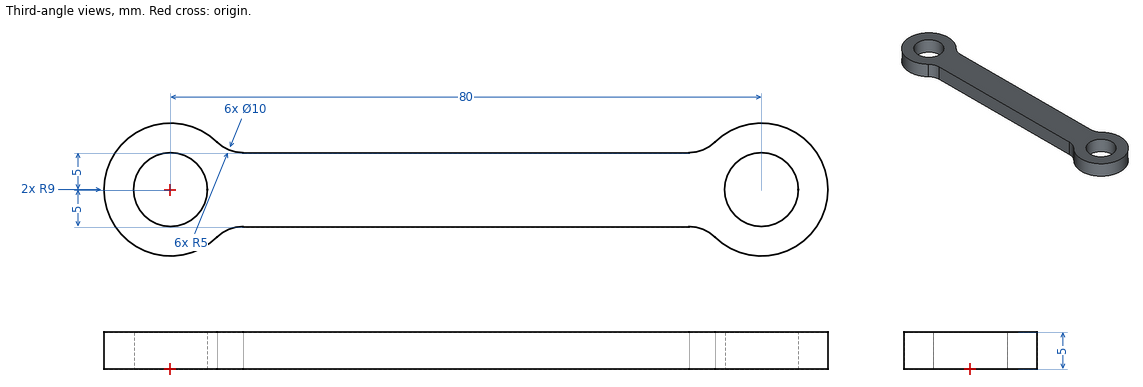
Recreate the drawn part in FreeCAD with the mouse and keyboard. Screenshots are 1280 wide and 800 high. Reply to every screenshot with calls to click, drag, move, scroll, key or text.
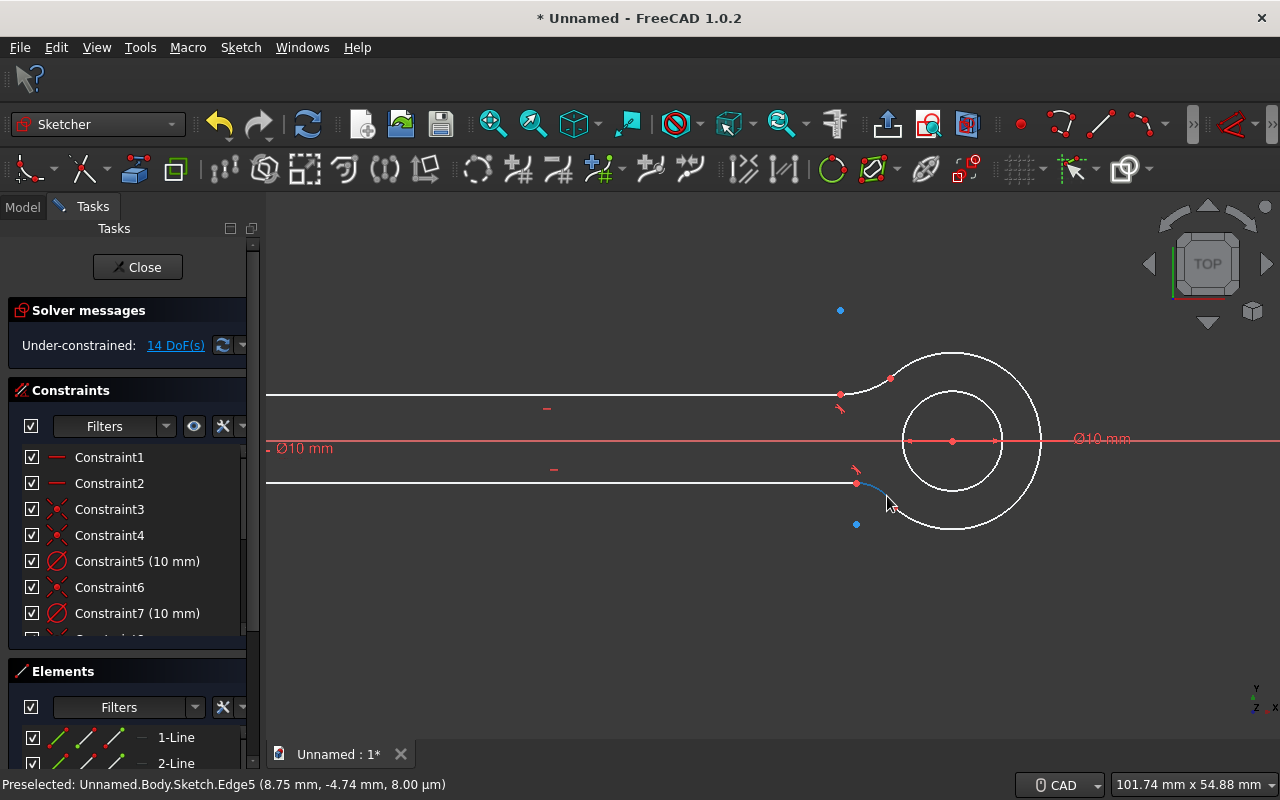
click(887, 496)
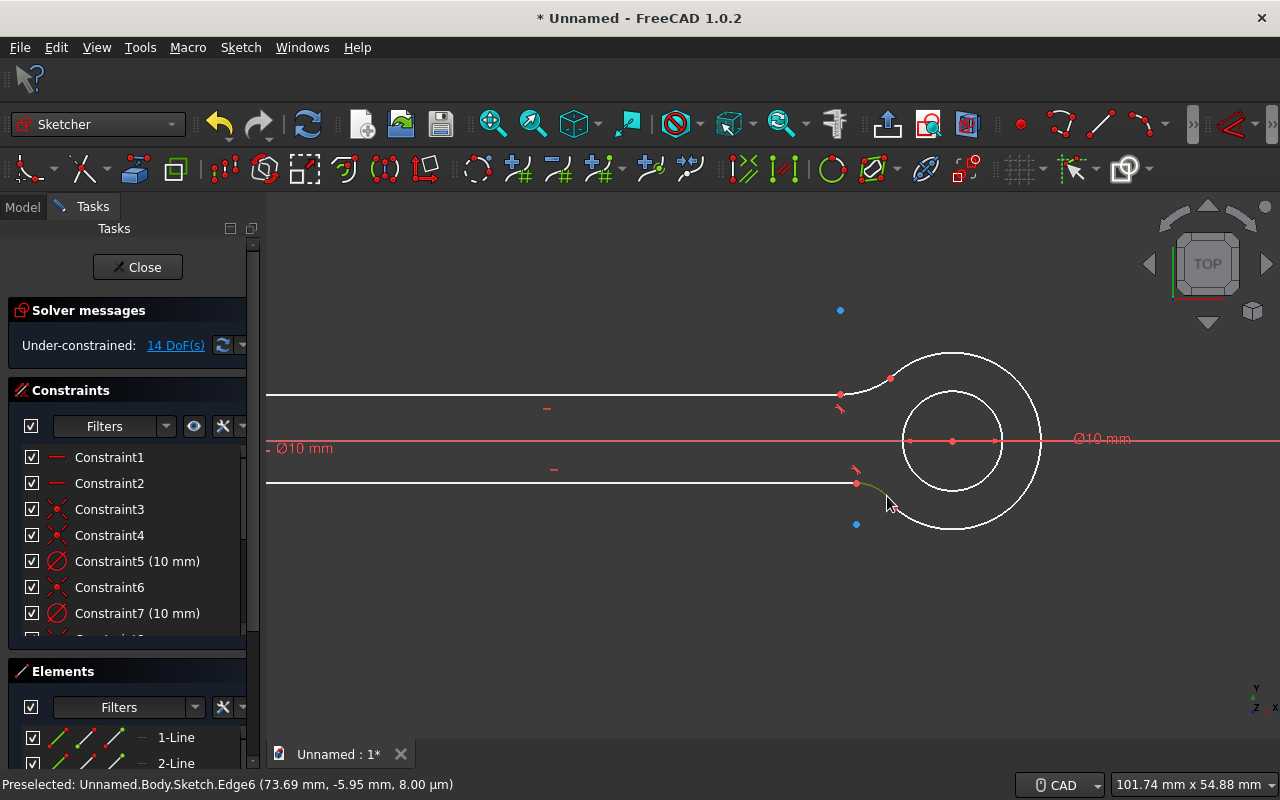
click(1008, 510)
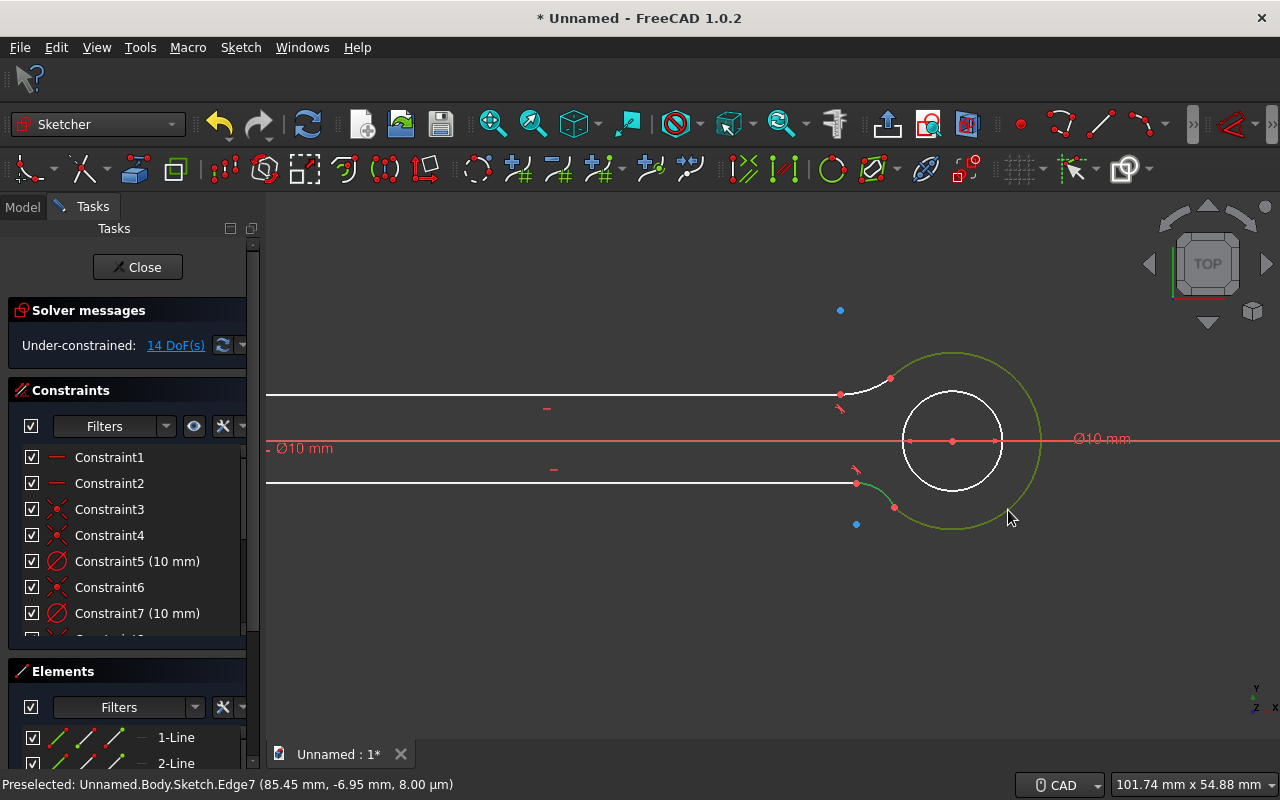
key(t)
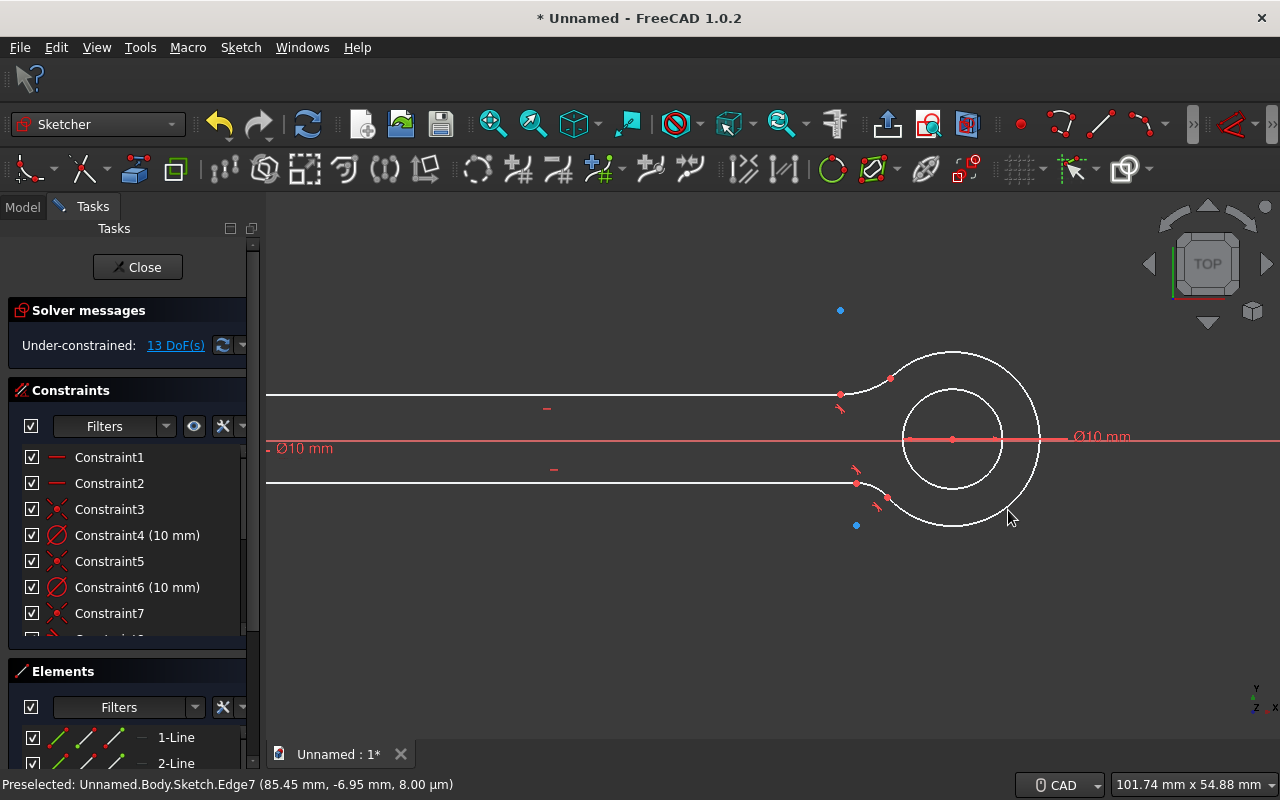
click(1001, 511)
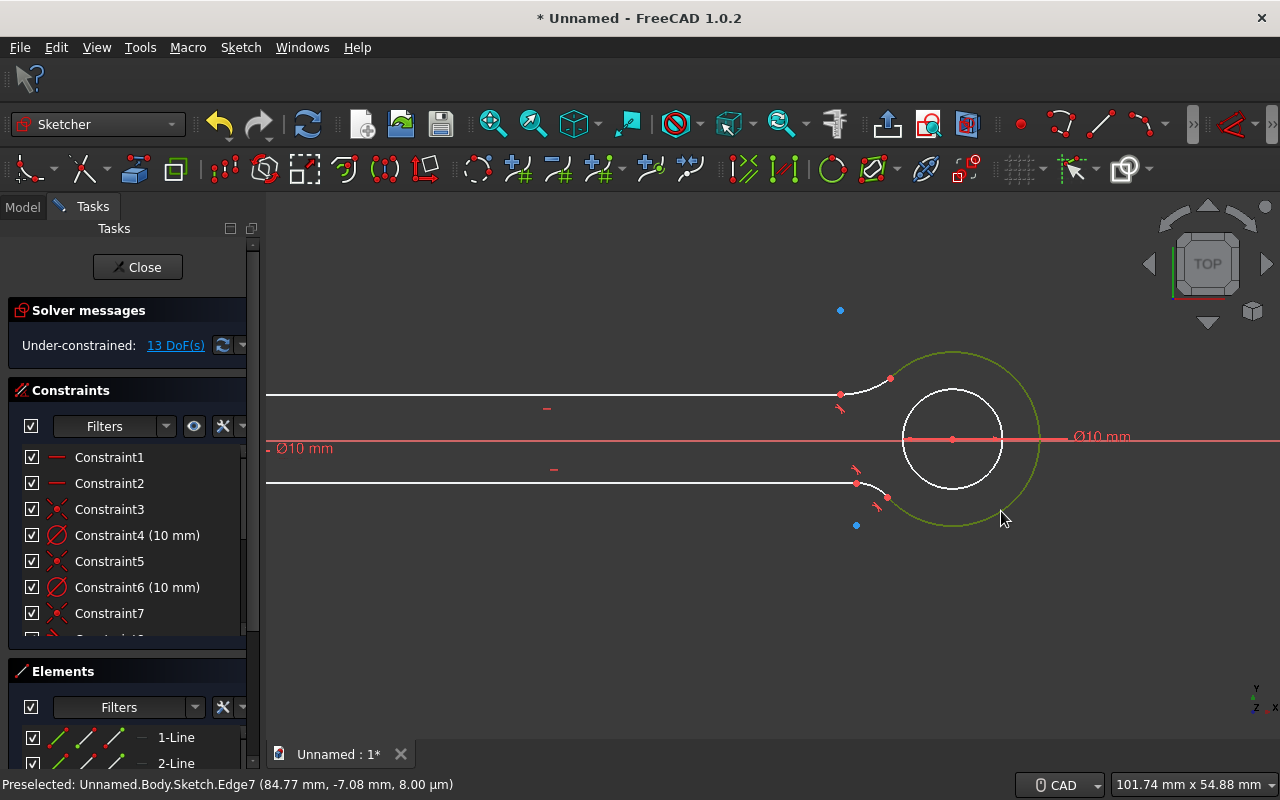
click(857, 393)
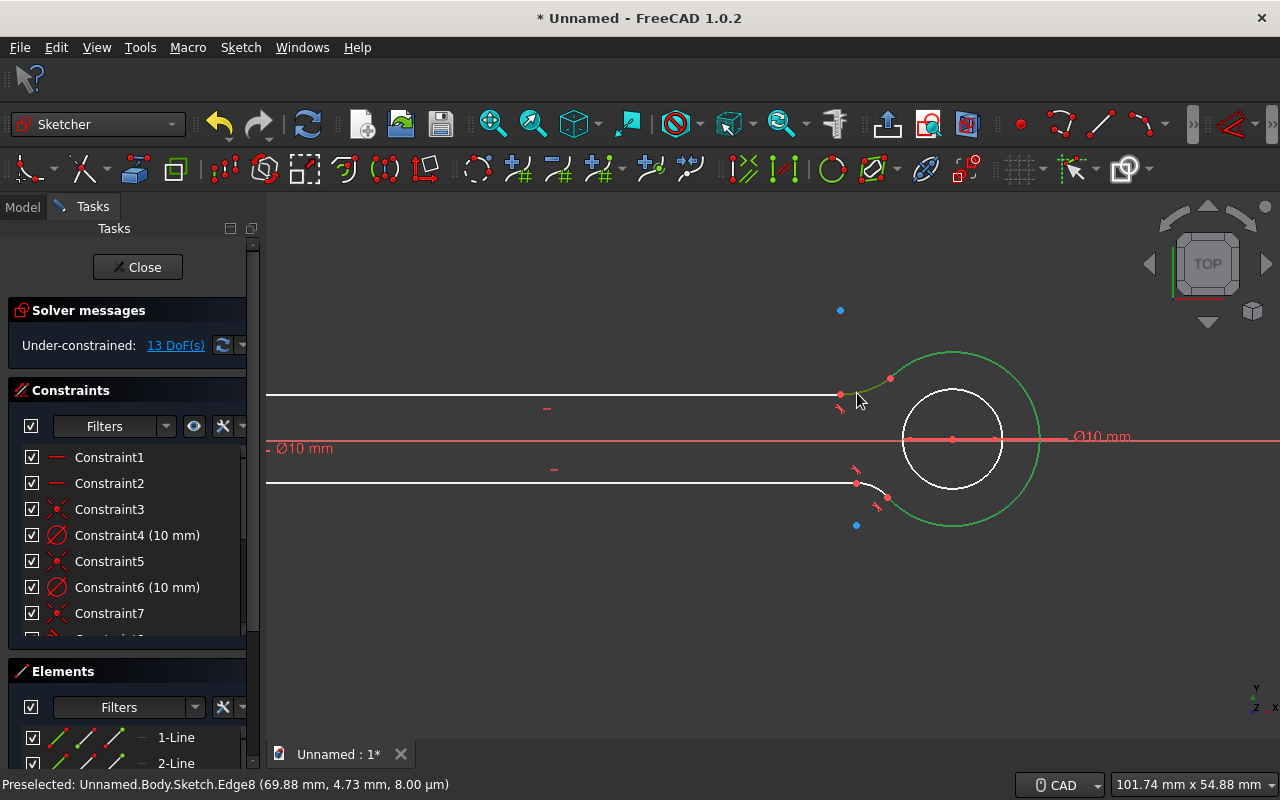
key(t)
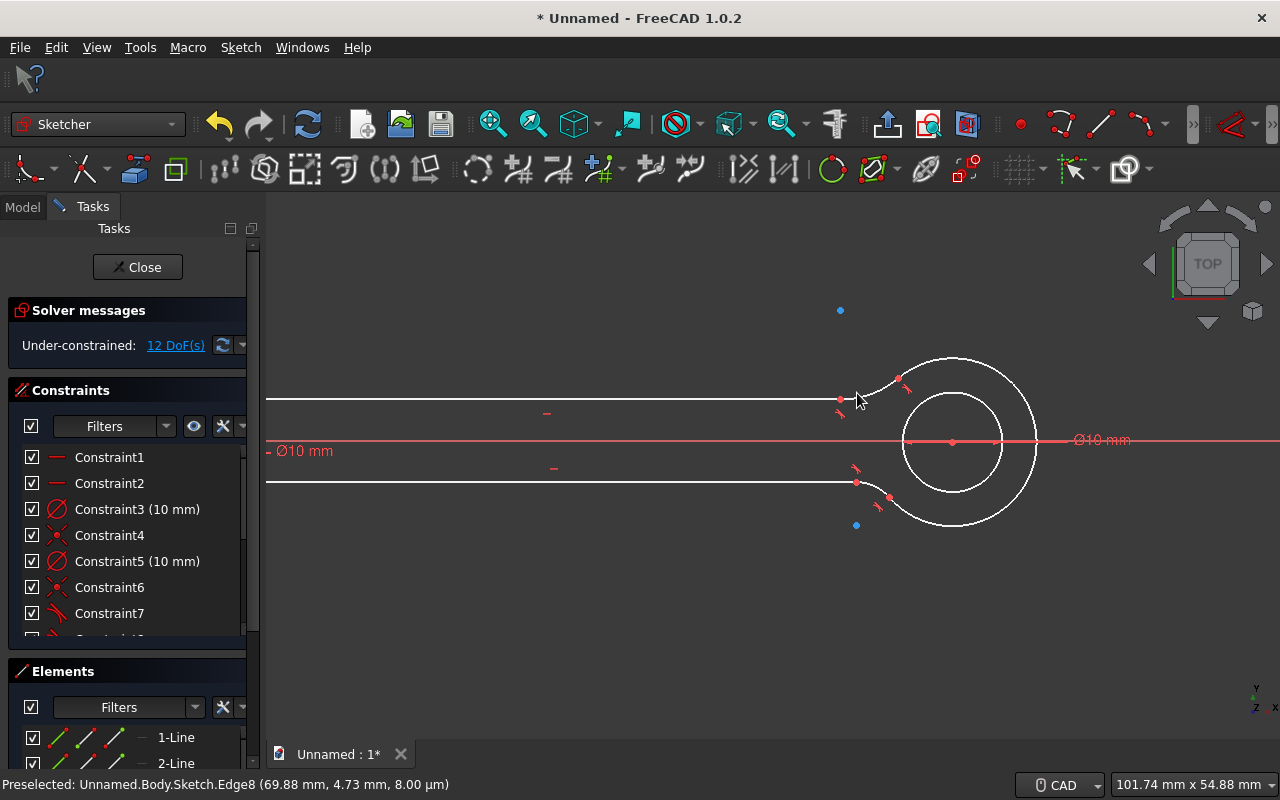
scroll(887, 495, down, 3)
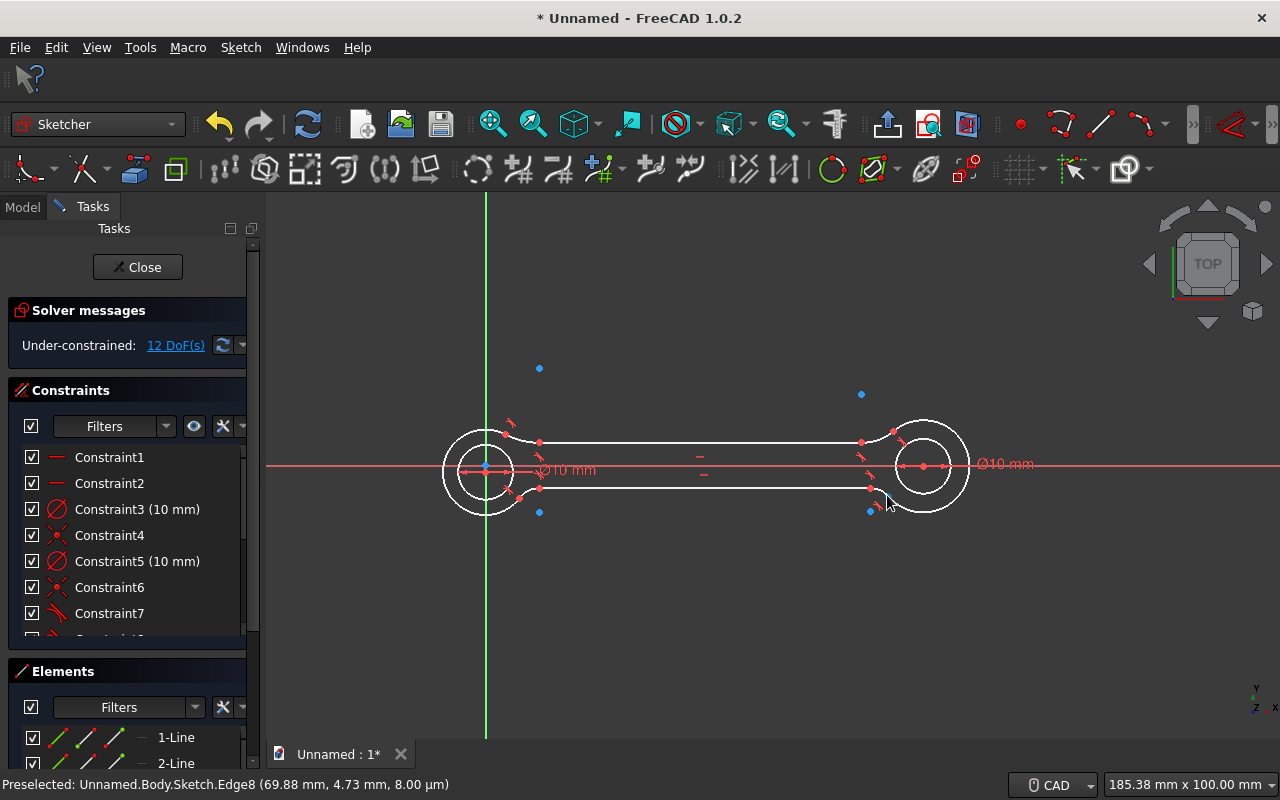
scroll(486, 469, up, 3)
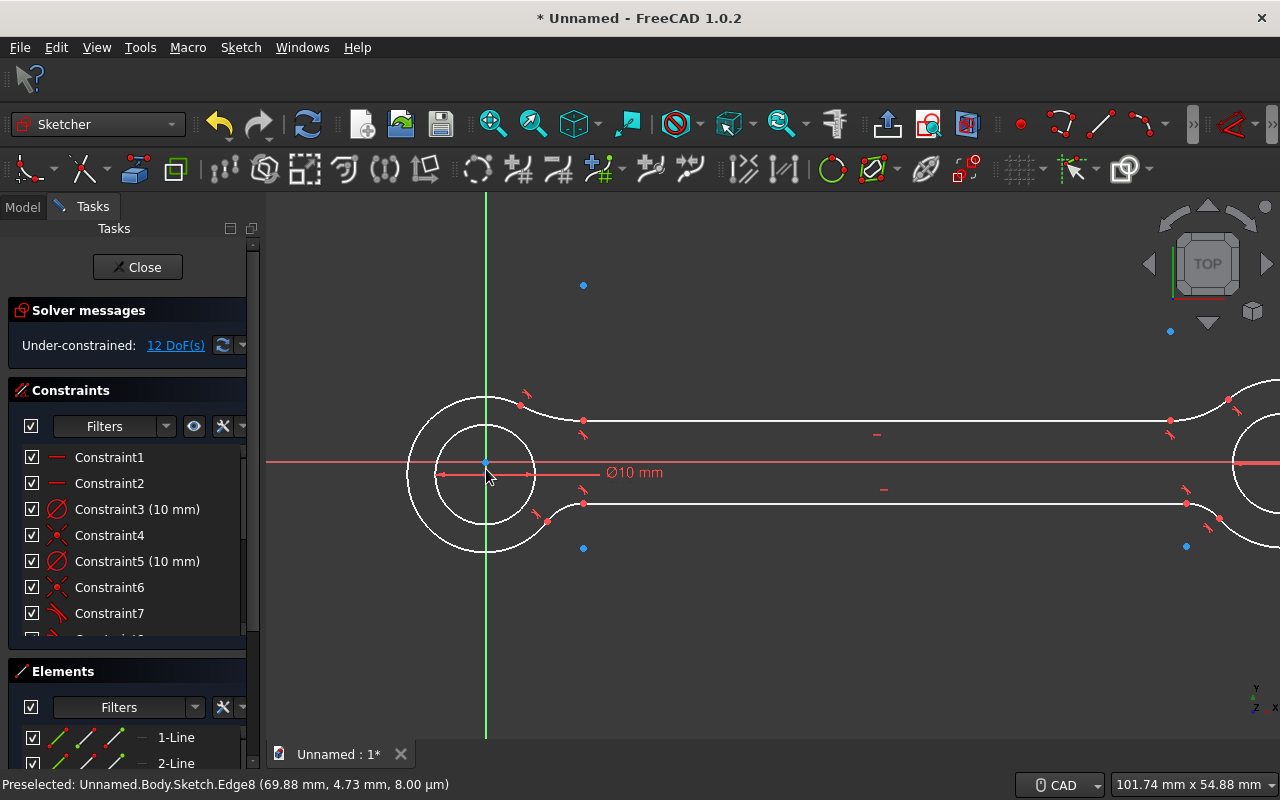
drag(475, 452, 496, 485)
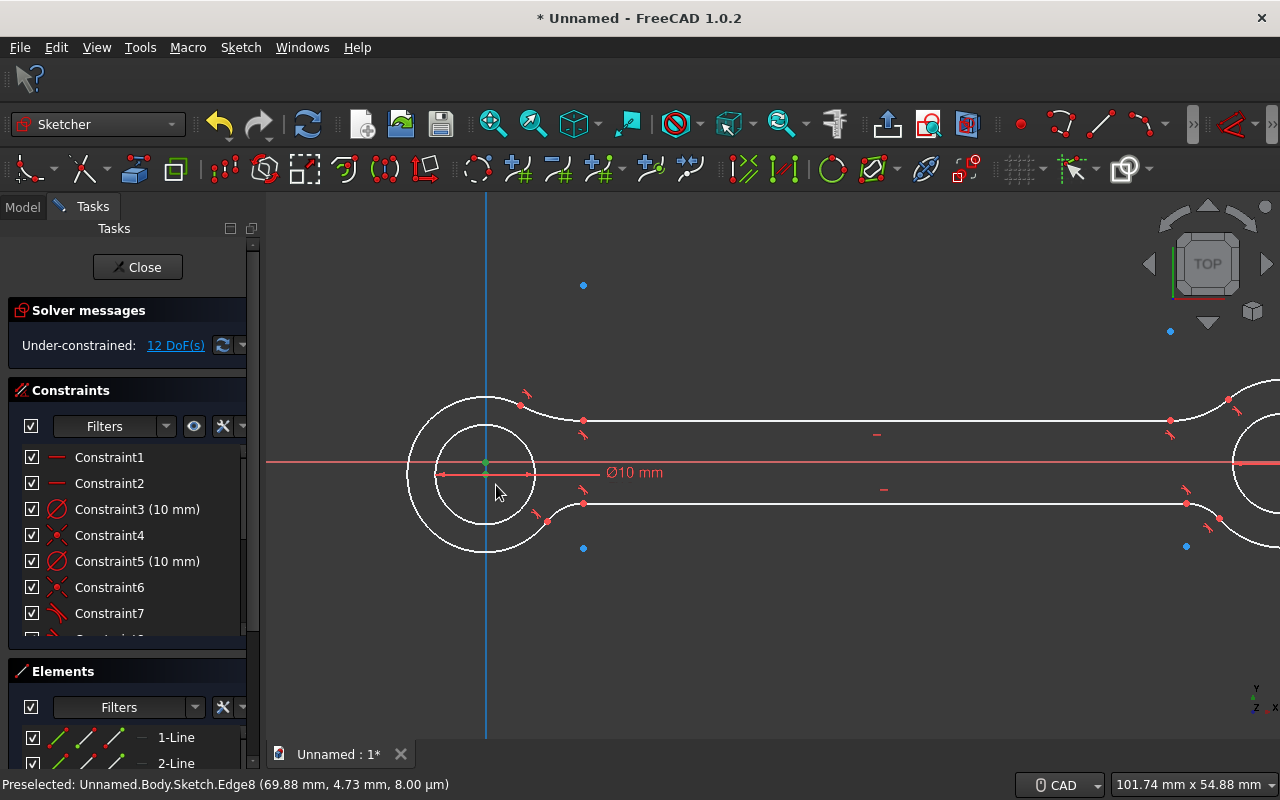
key(c)